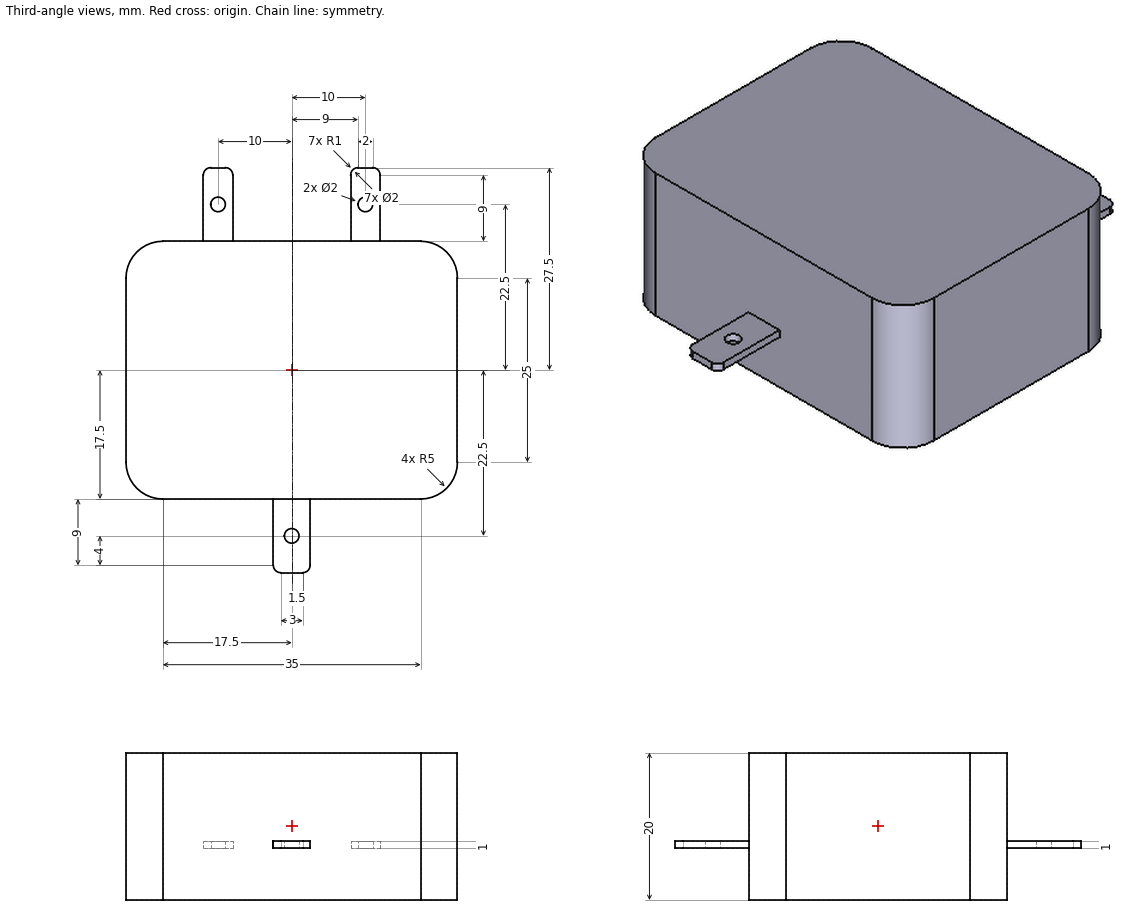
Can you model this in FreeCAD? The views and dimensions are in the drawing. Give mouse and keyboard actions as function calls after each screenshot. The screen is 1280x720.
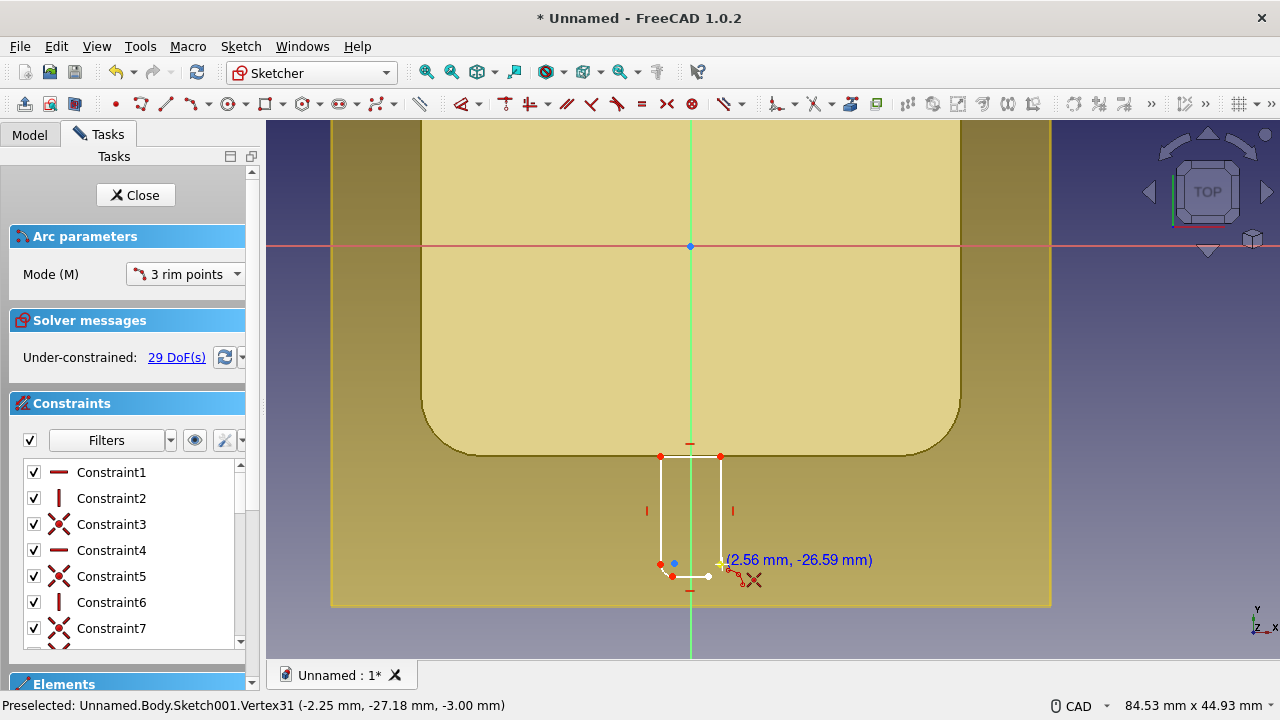
click(721, 565)
click(709, 577)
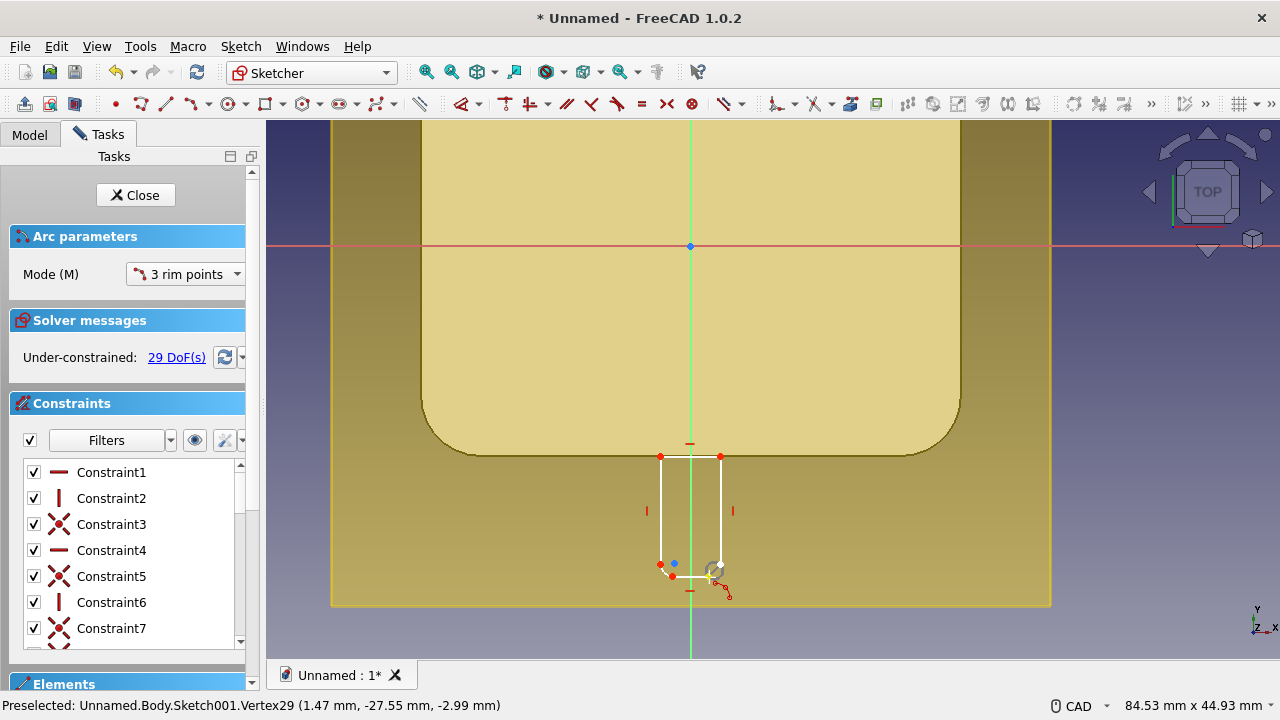
scroll(717, 573, up, 8)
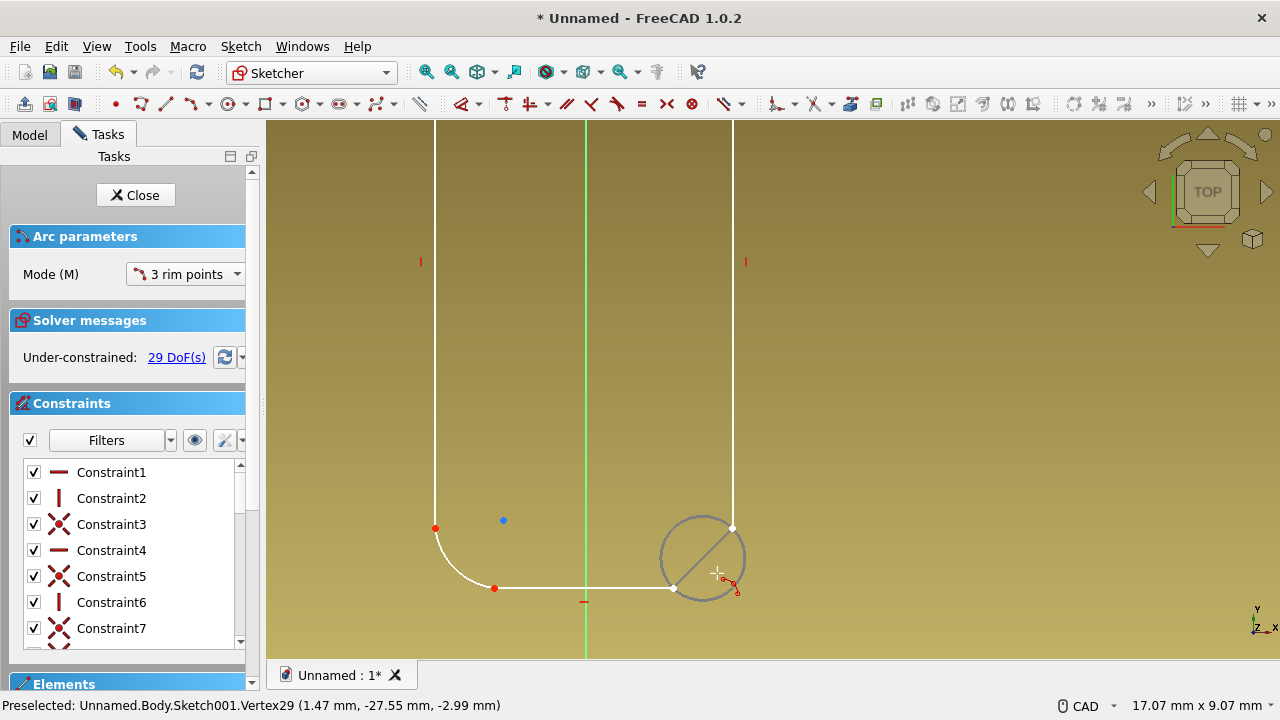
click(717, 567)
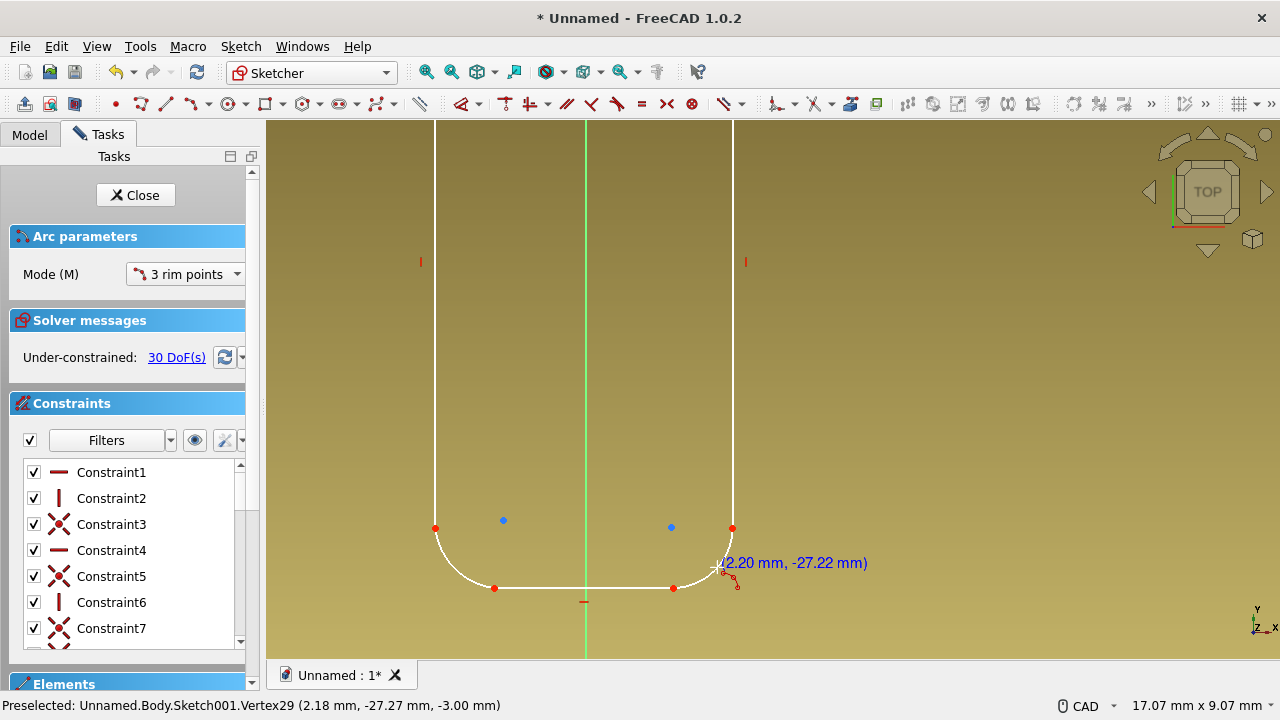
click(228, 104)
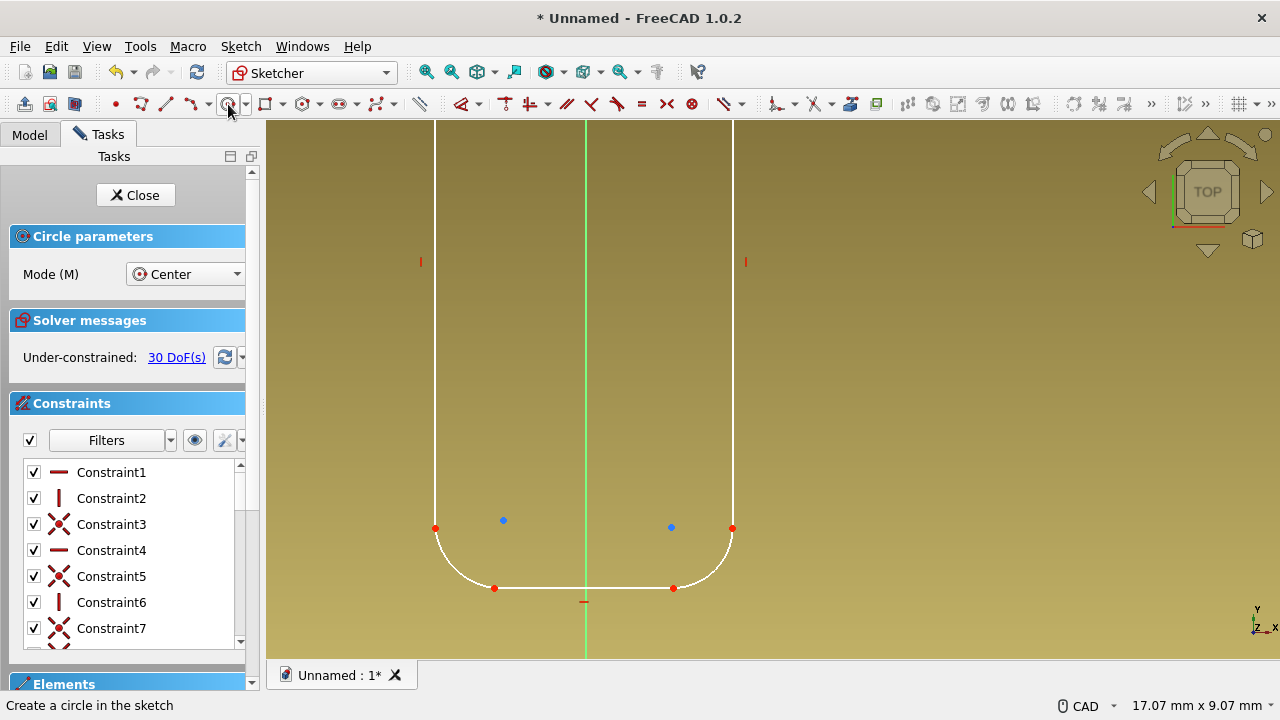
scroll(719, 569, down, 11)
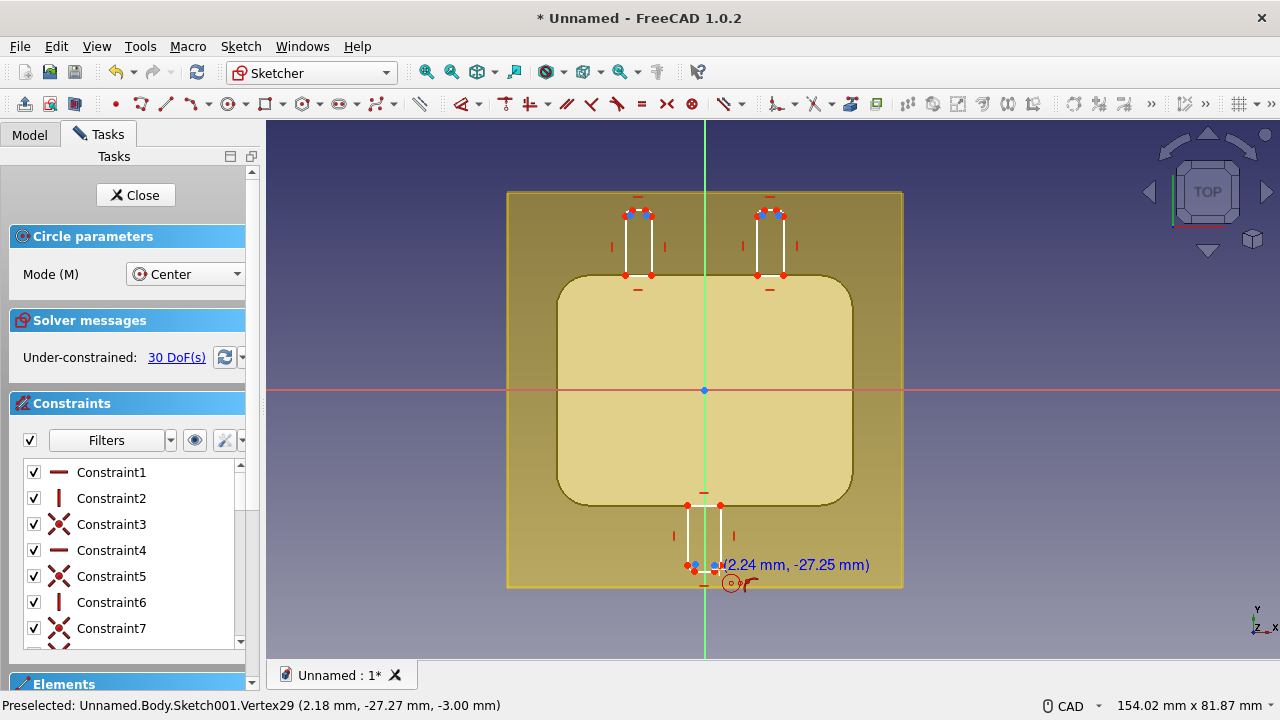
click(705, 539)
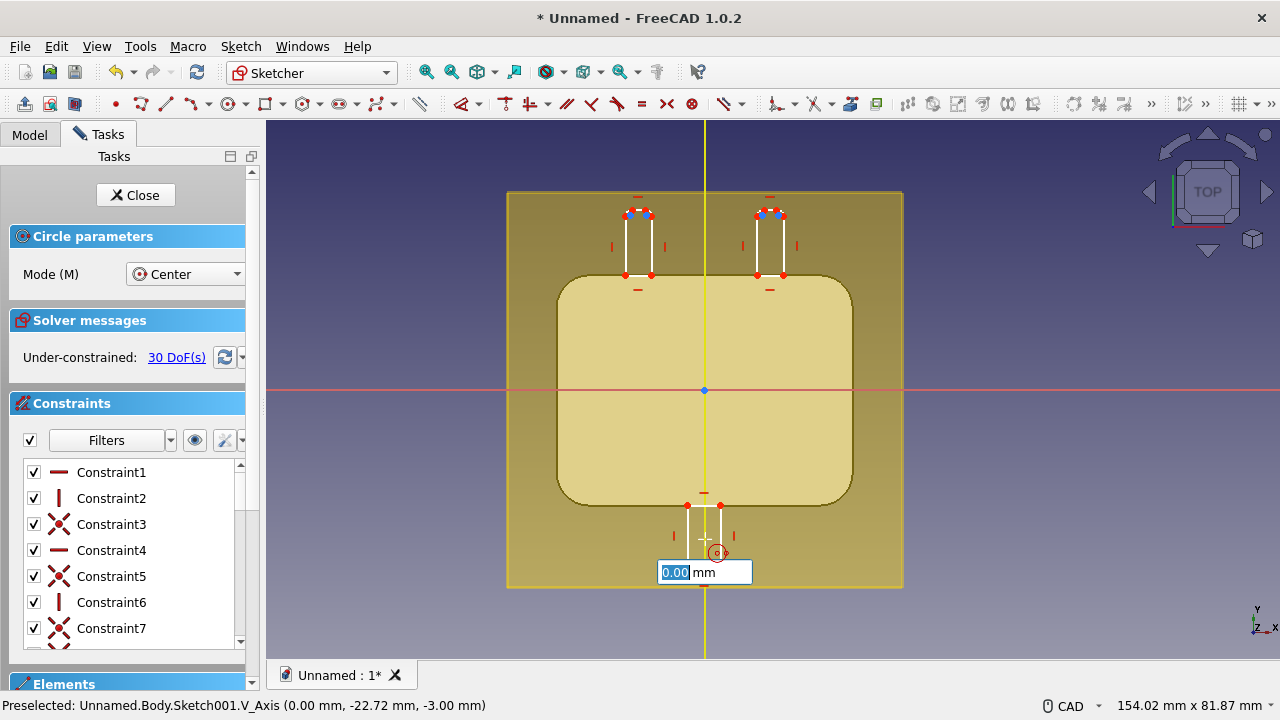
scroll(711, 536, up, 5)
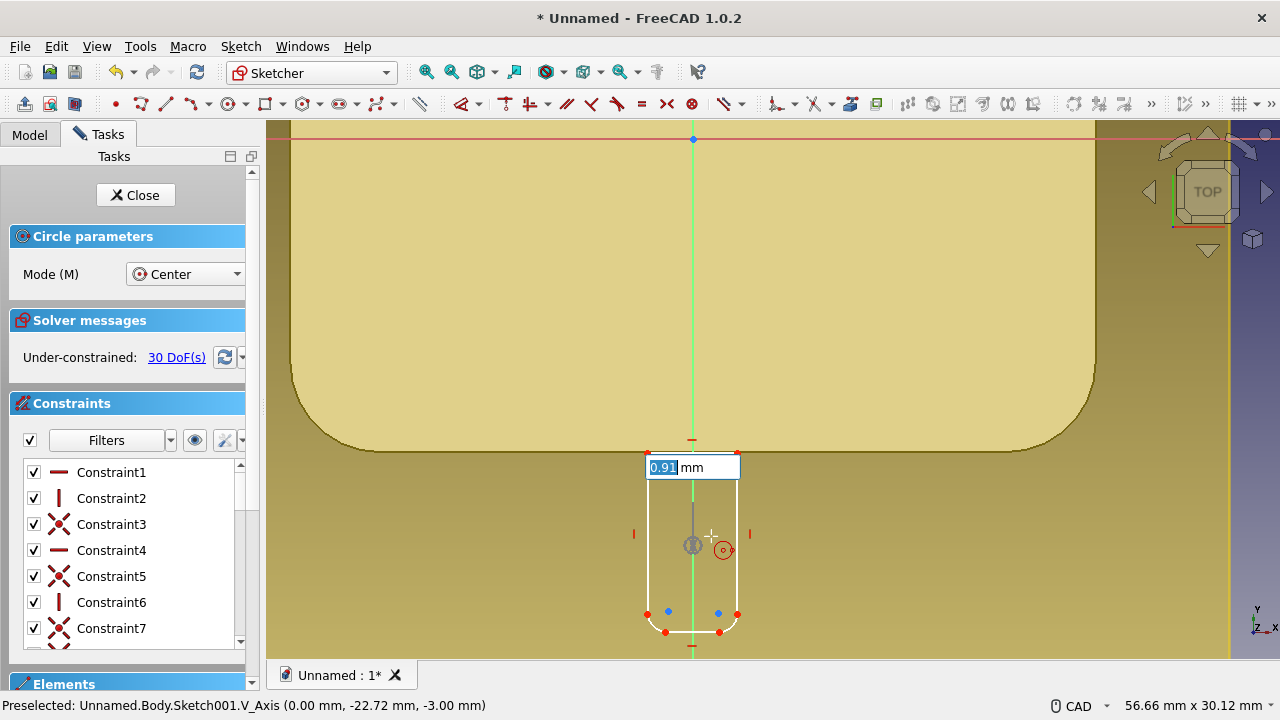
click(710, 536)
key(Escape)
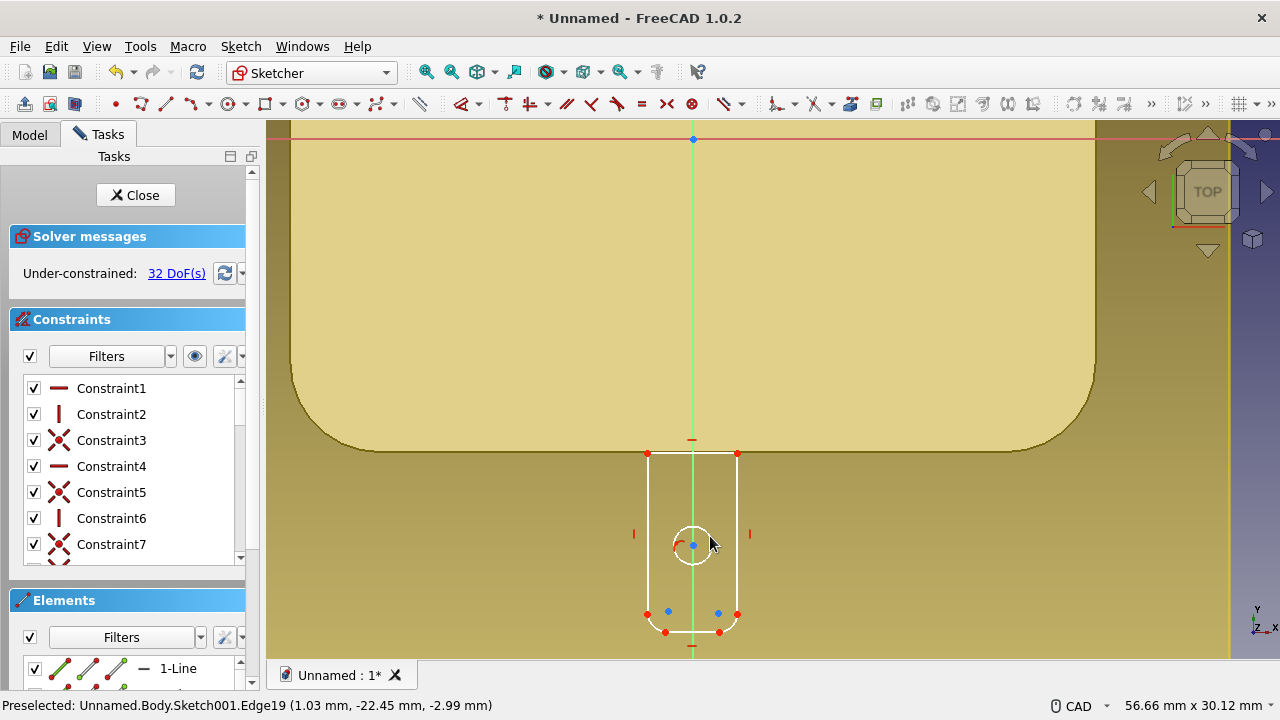
scroll(711, 535, down, 5)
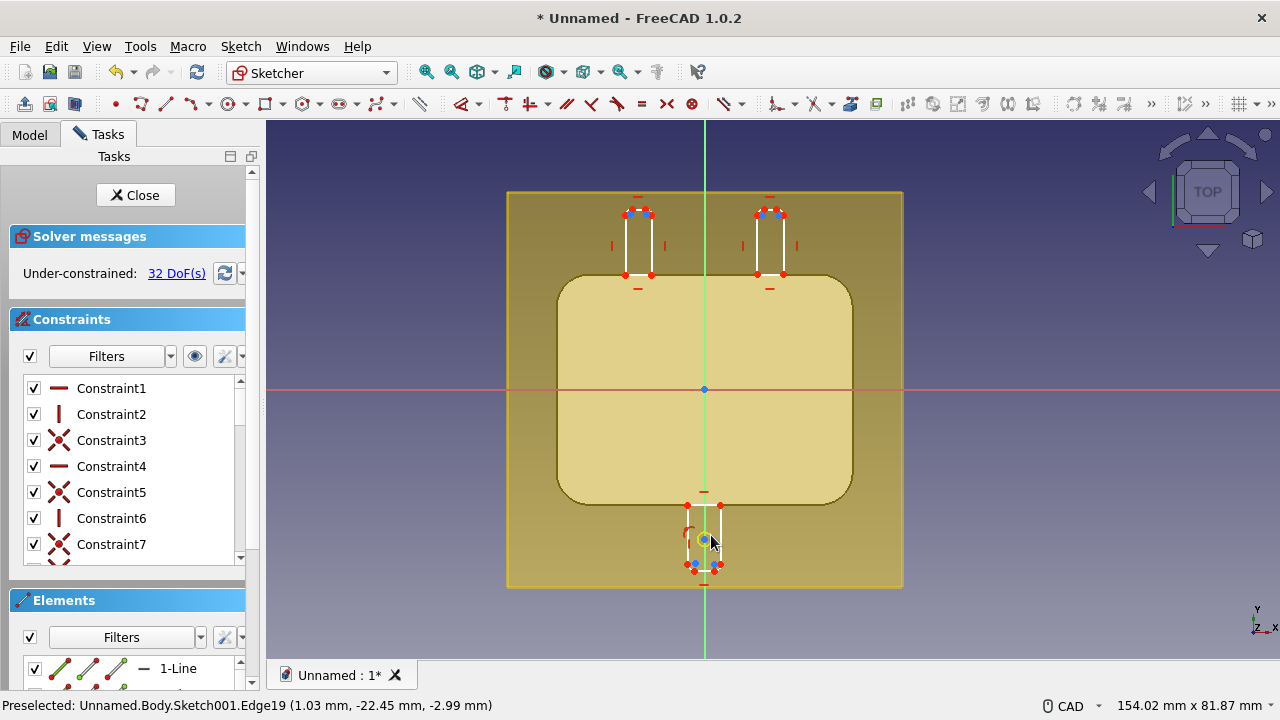
scroll(768, 210, up, 7)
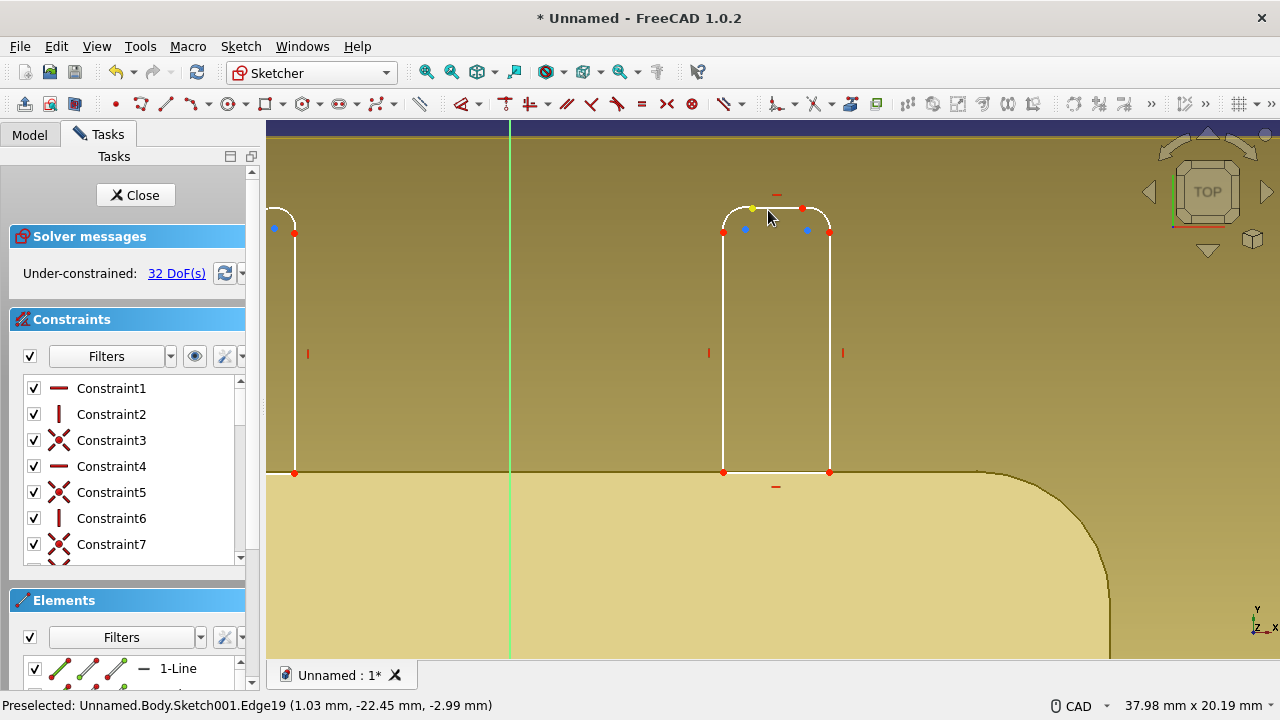
click(767, 208)